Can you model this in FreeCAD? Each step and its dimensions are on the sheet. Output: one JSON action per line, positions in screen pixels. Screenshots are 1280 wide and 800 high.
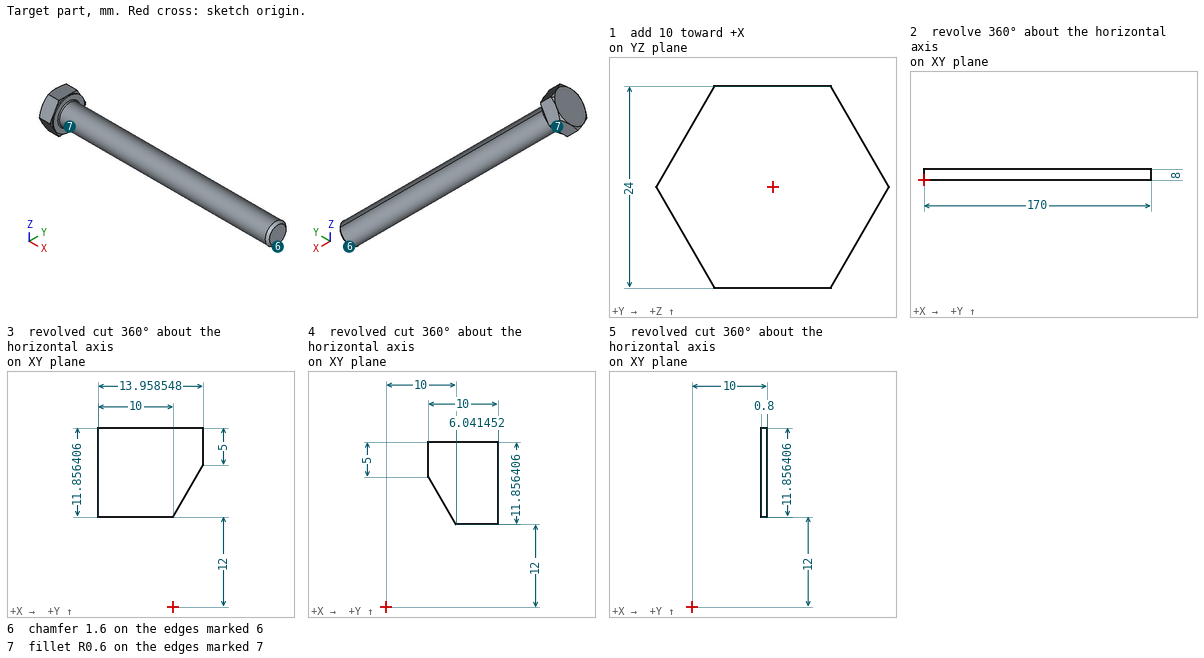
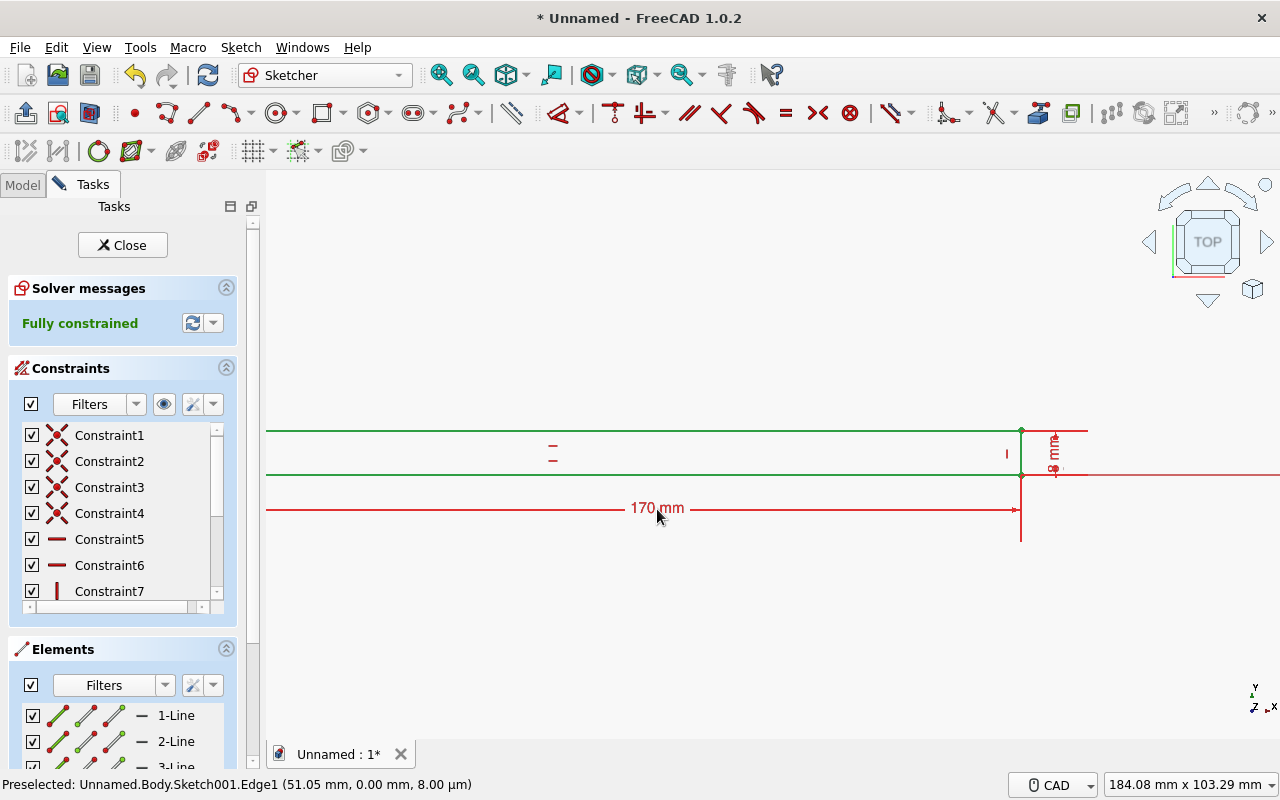
{"action": "left_click", "coordinate": [123, 245]}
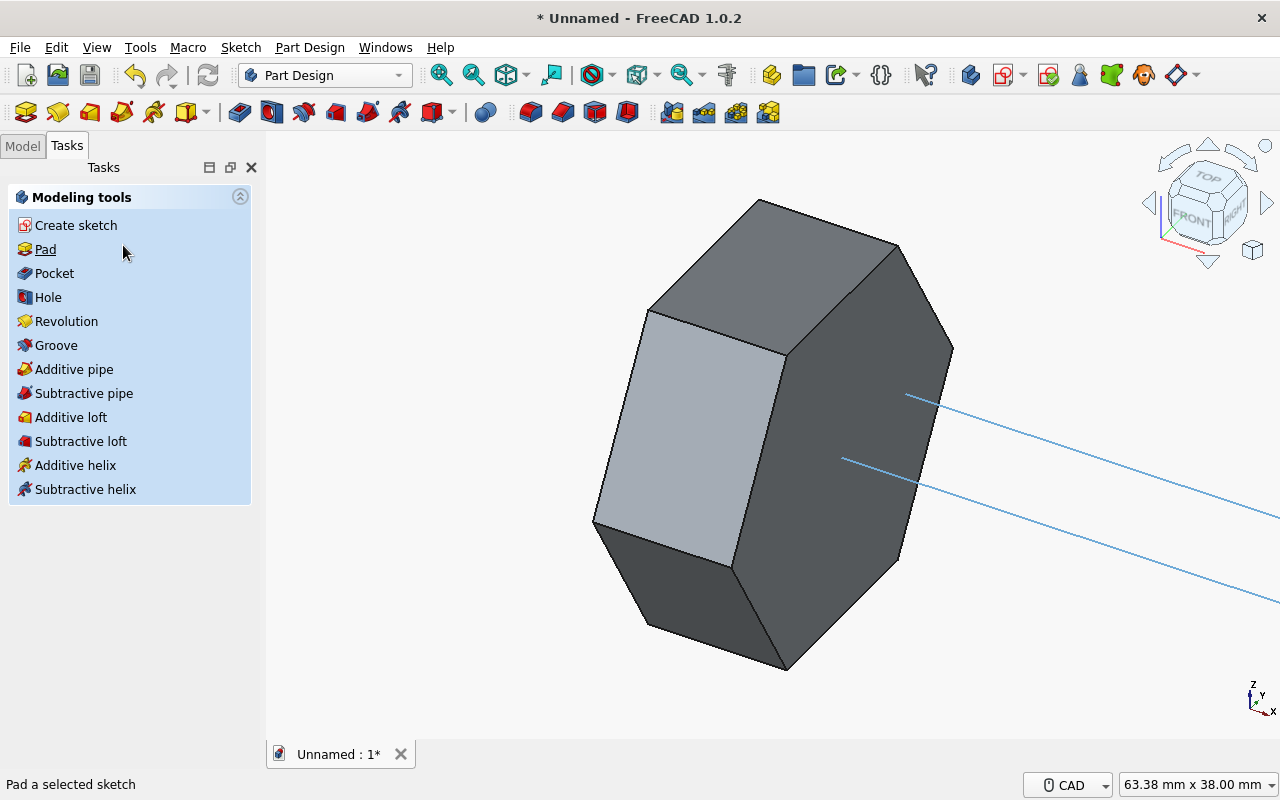
{"action": "left_click", "coordinate": [58, 112]}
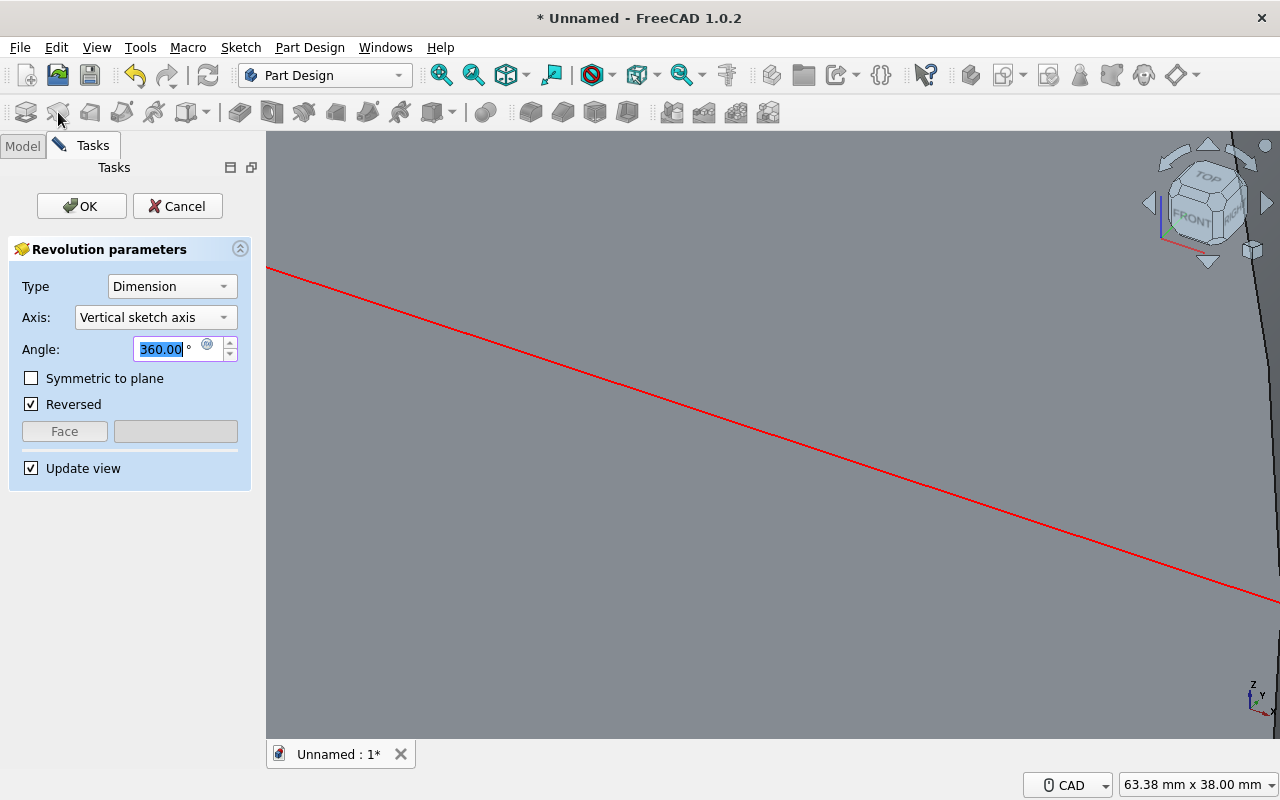
{"action": "left_click", "coordinate": [156, 318]}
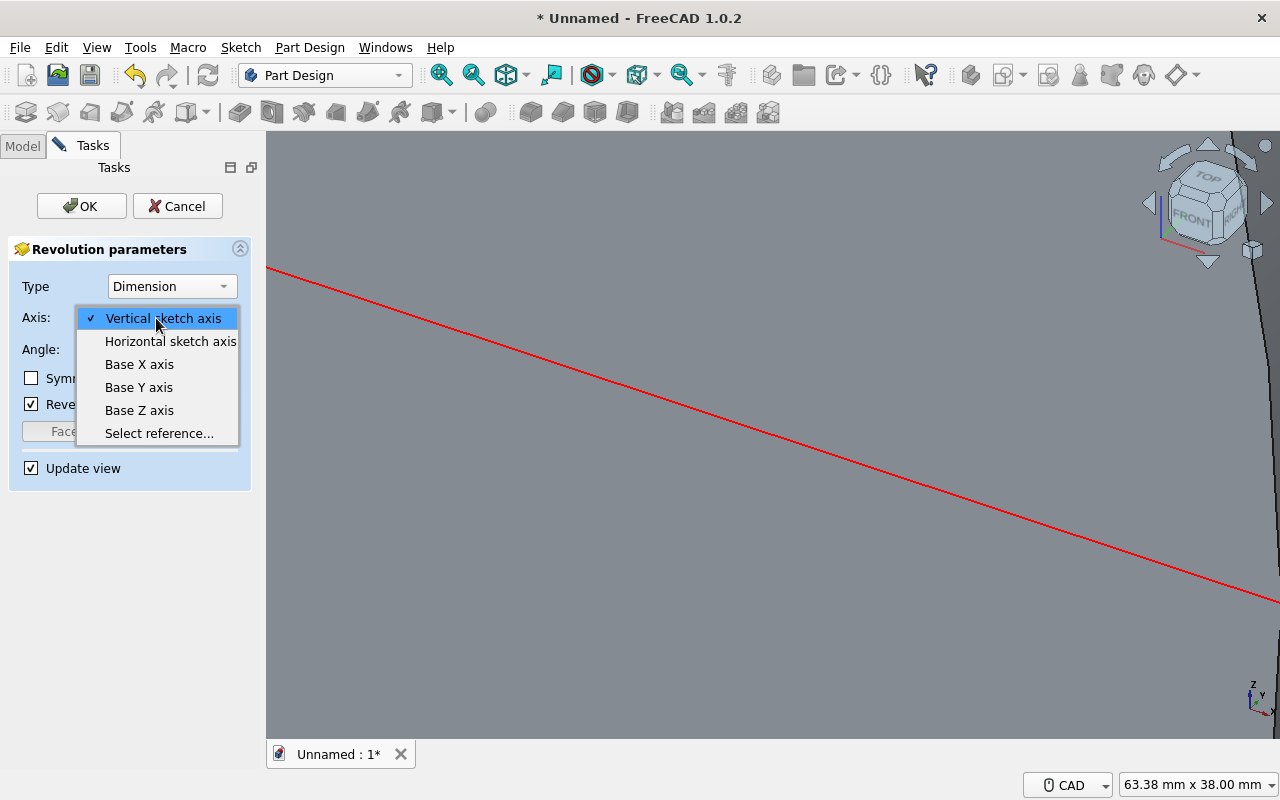
{"action": "left_click", "coordinate": [156, 342]}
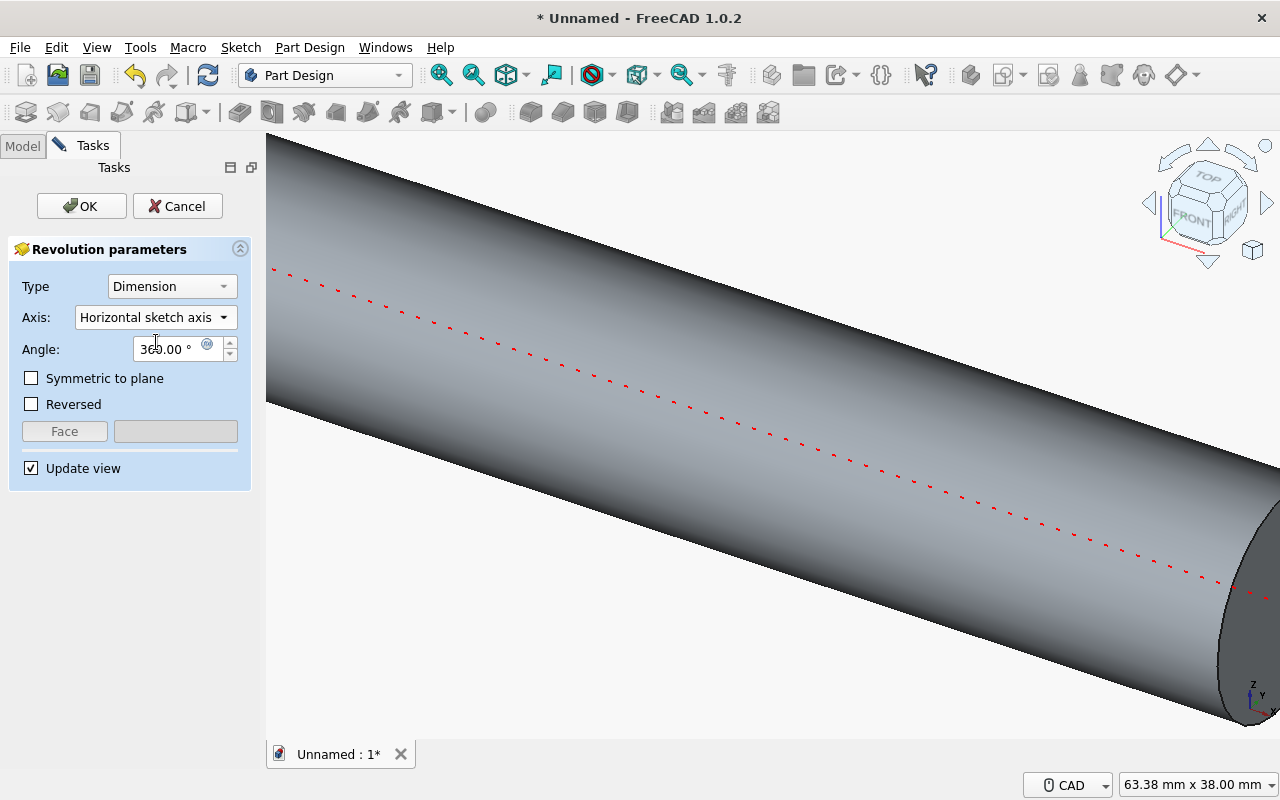
{"action": "left_click", "coordinate": [82, 206]}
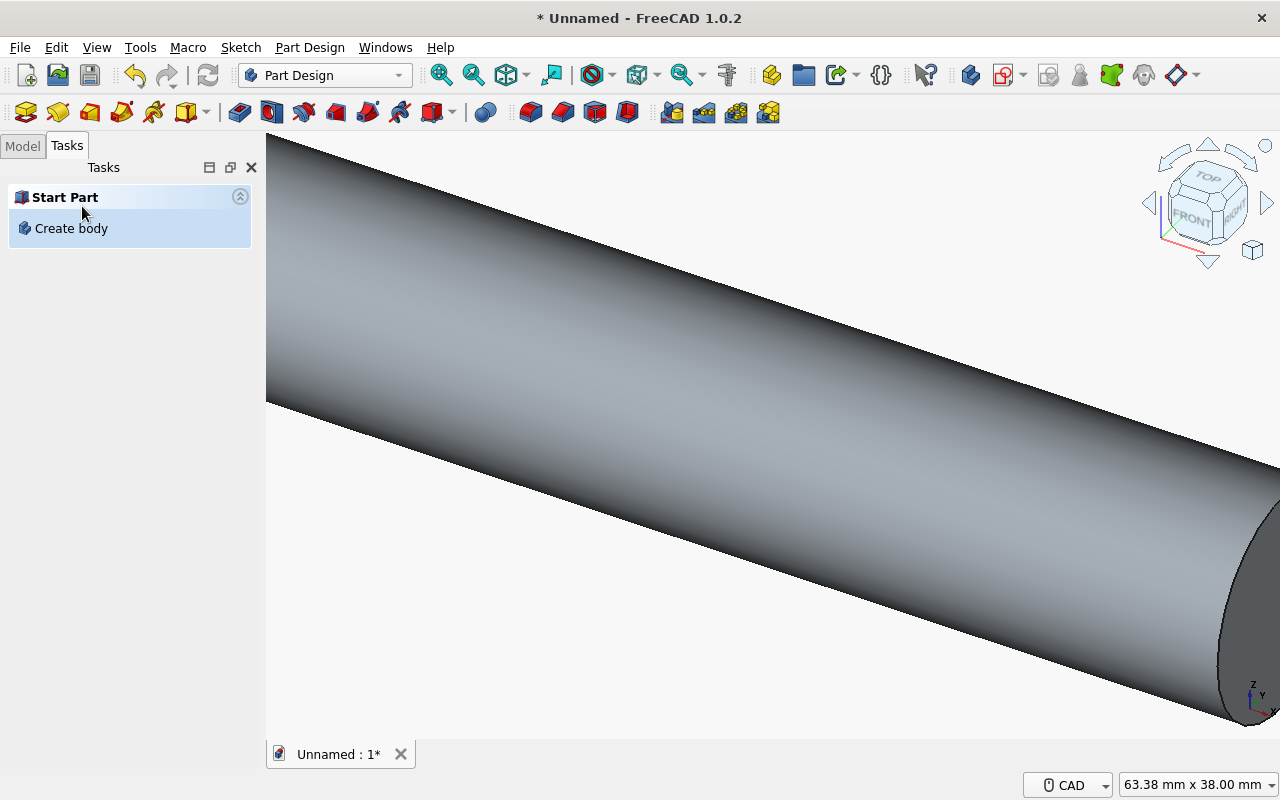
{"action": "left_click", "coordinate": [442, 76]}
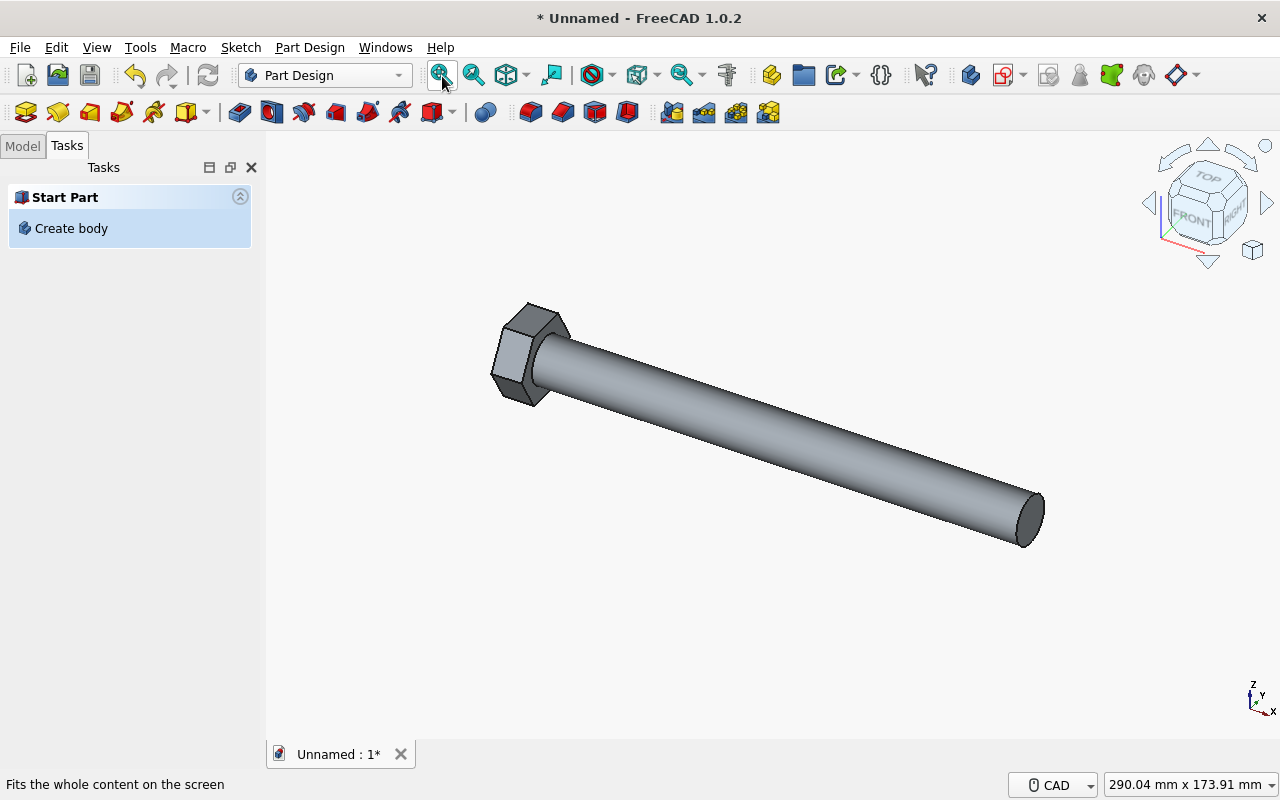
{"action": "left_click", "coordinate": [1004, 76]}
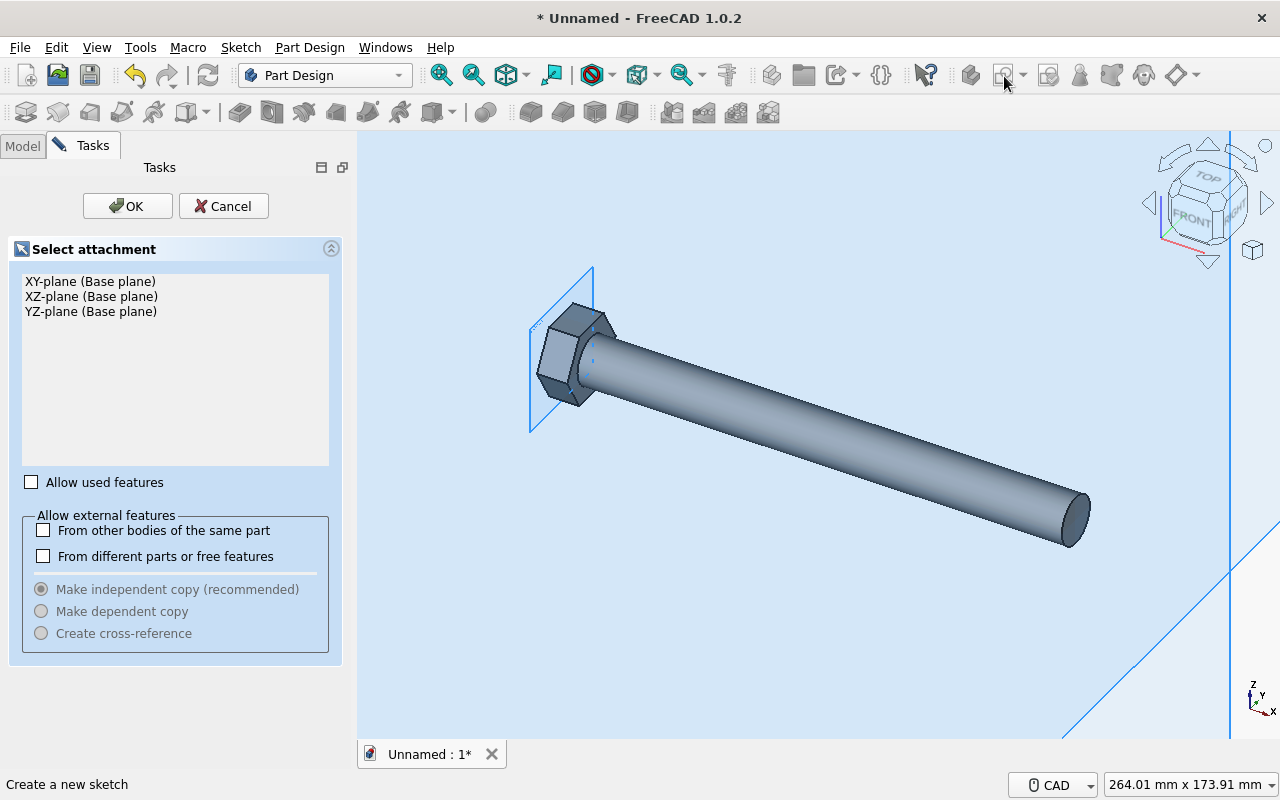
{"action": "left_click", "coordinate": [82, 282]}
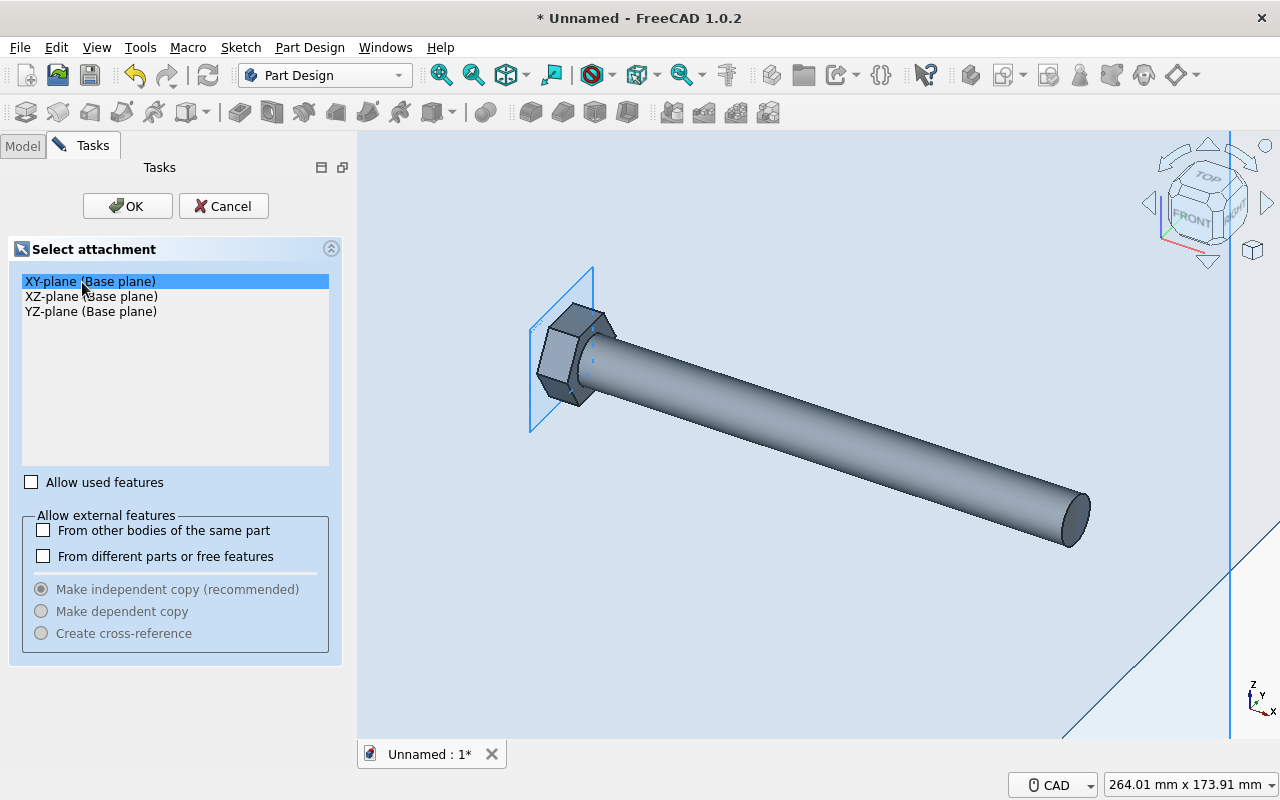
{"action": "left_click", "coordinate": [128, 206]}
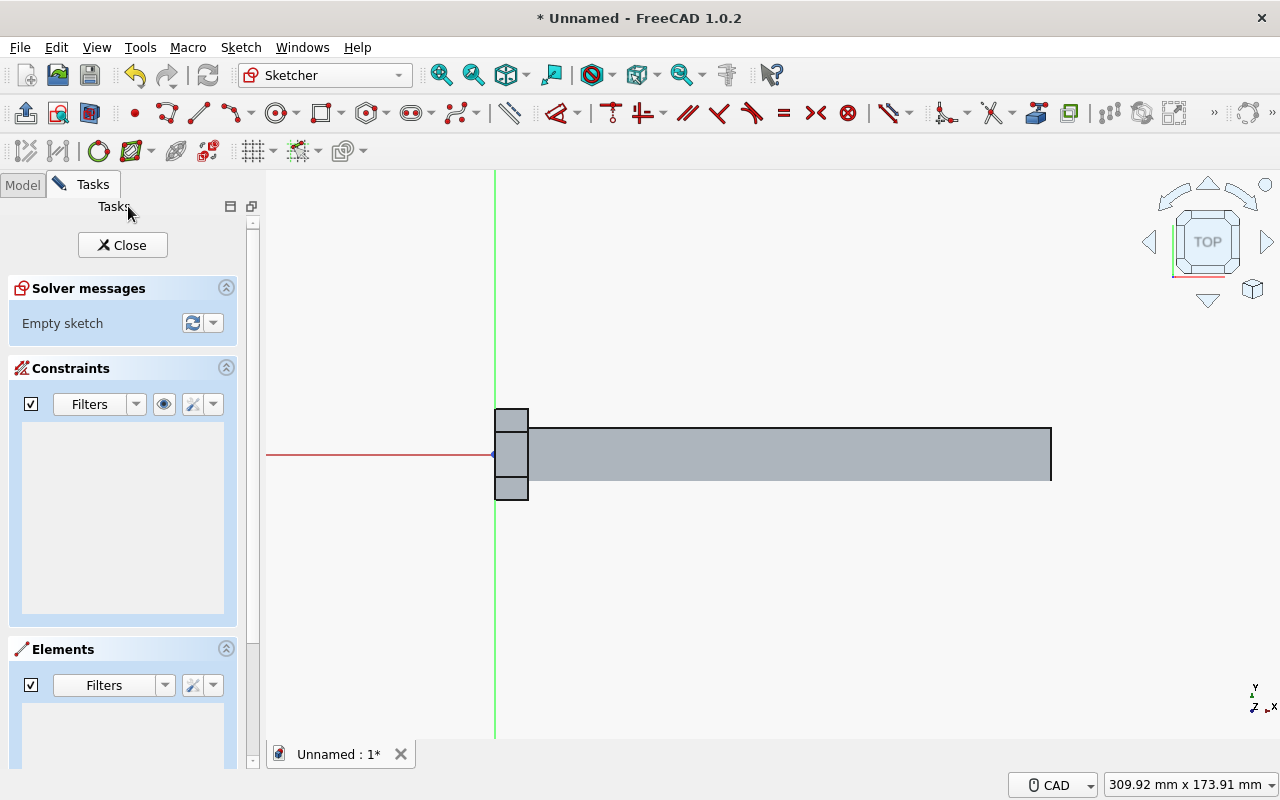
{"action": "left_click", "coordinate": [90, 114]}